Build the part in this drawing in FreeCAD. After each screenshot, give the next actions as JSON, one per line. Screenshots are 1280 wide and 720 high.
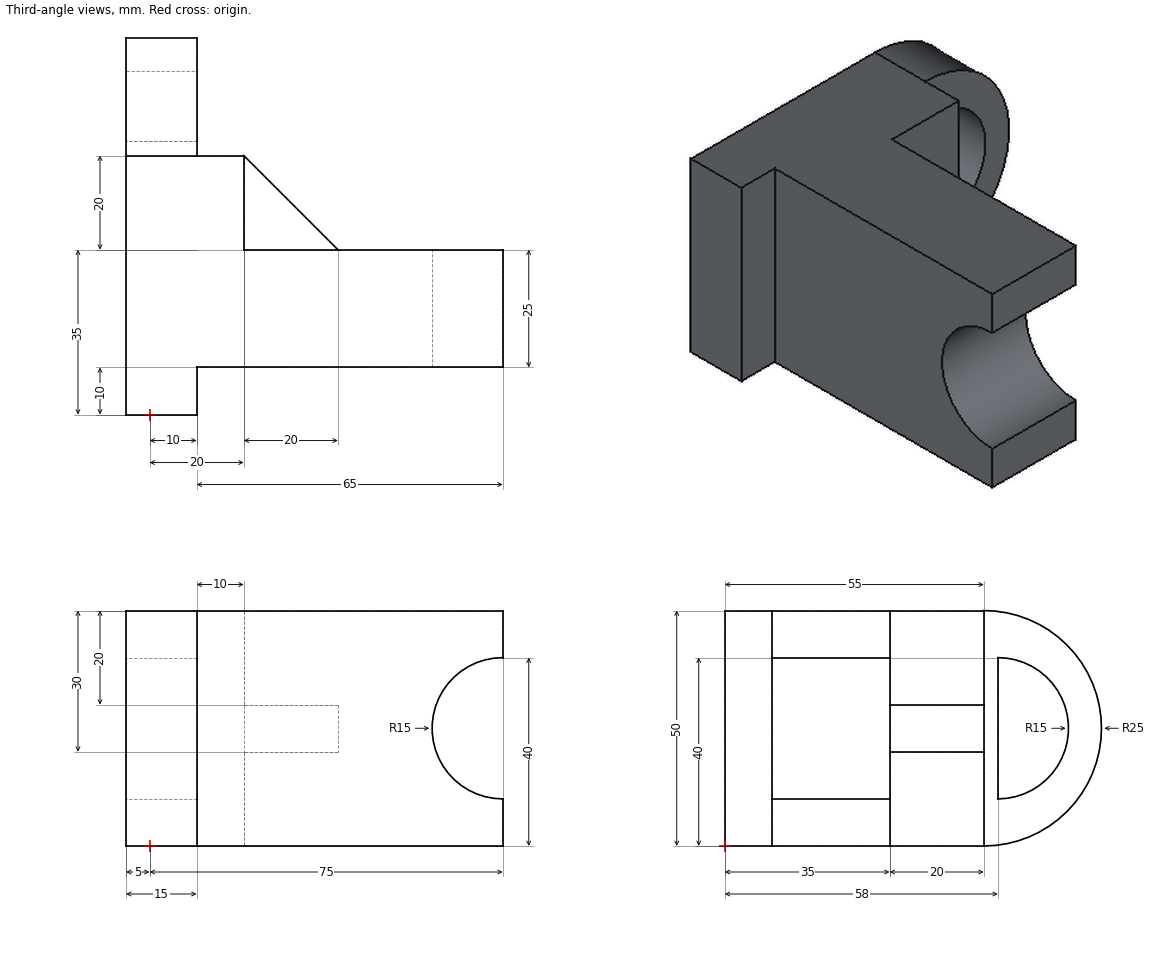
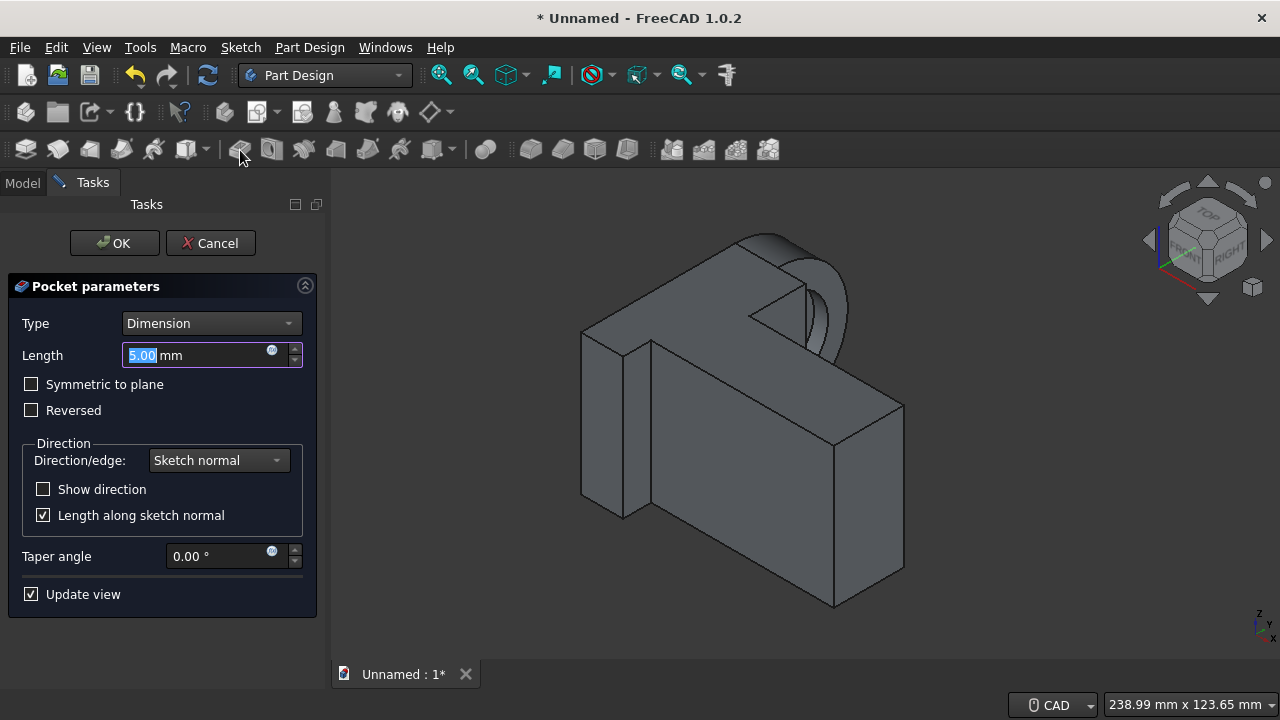
{"action": "type", "text": "15"}
{"action": "key", "text": "Tab"}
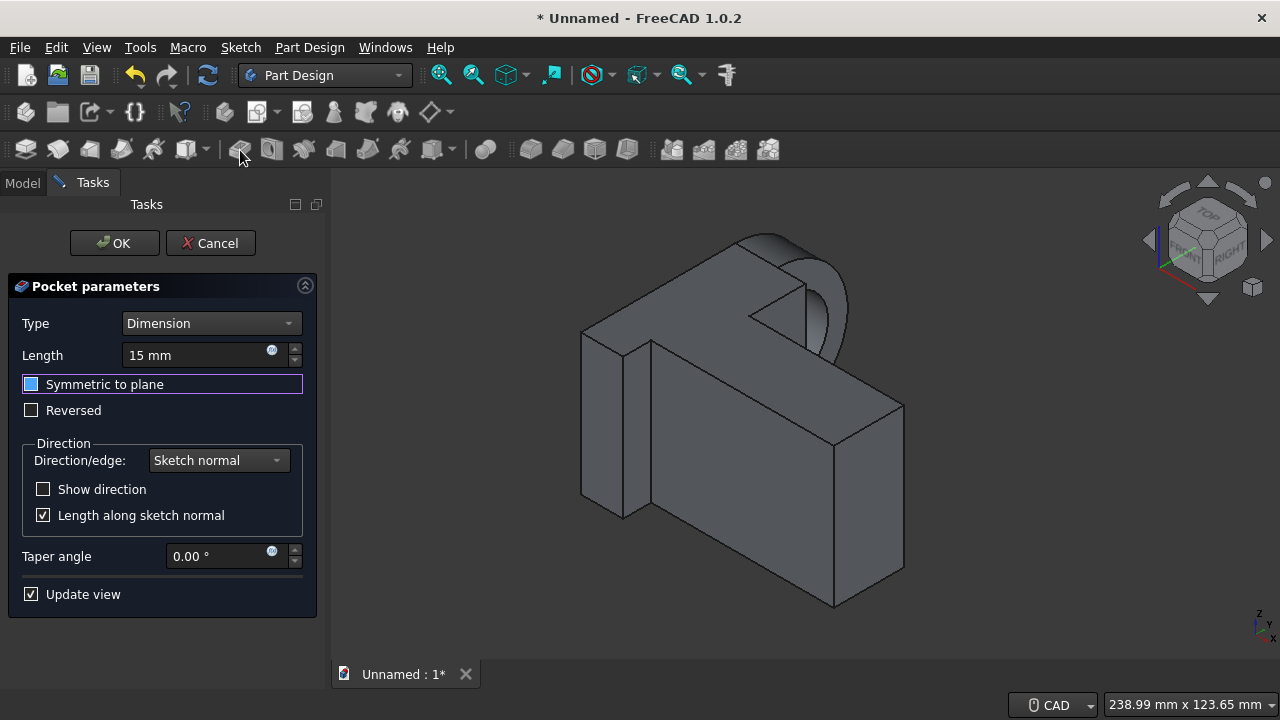
{"action": "left_click", "coordinate": [115, 243]}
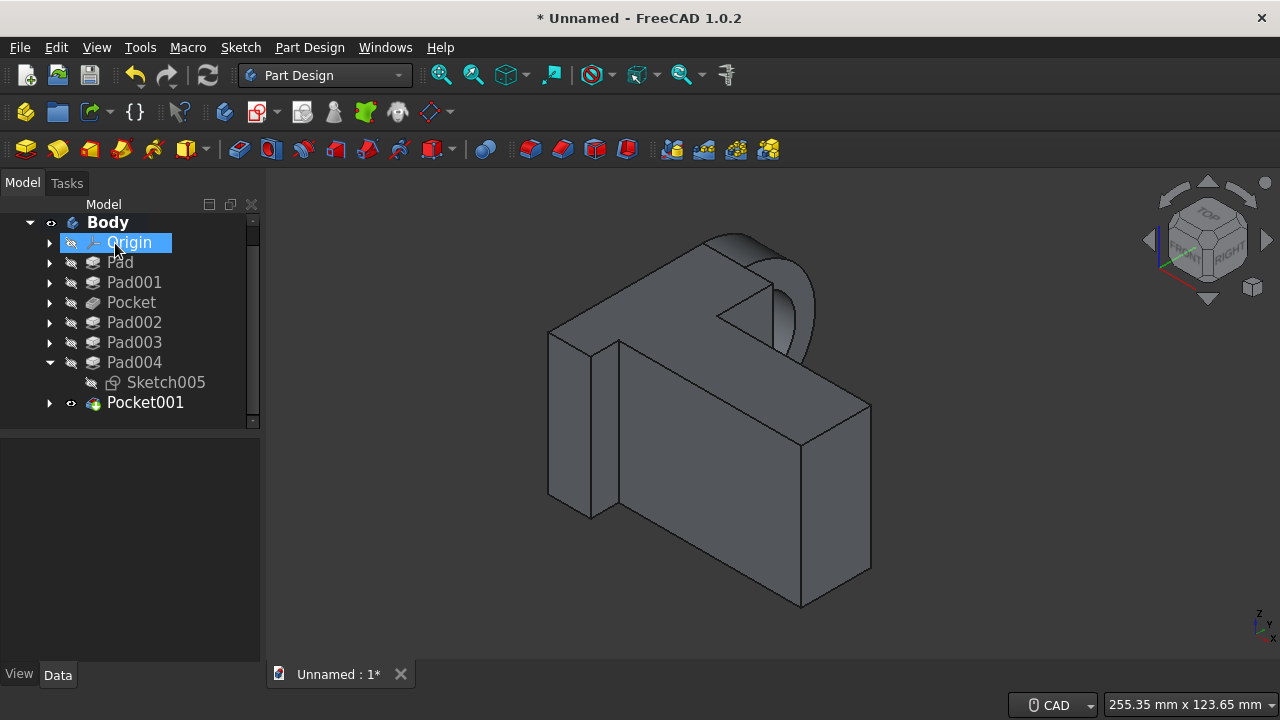
{"action": "key", "text": "4"}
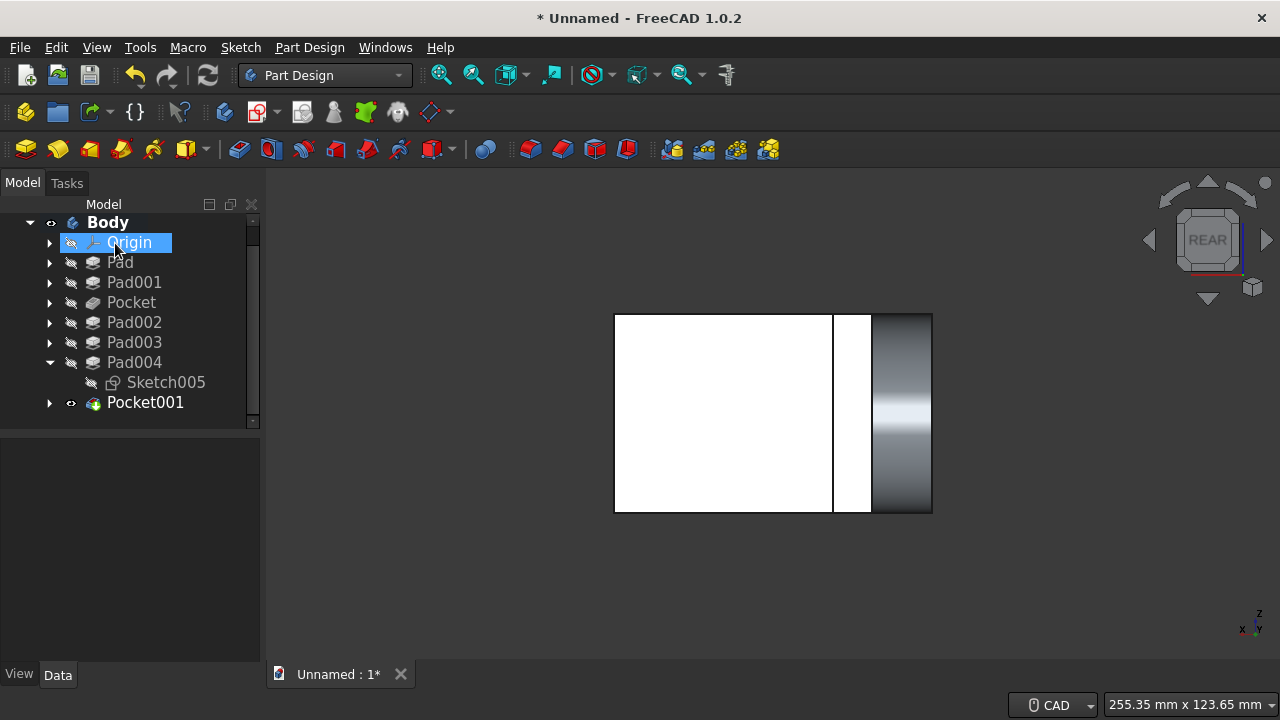
{"action": "left_click", "coordinate": [442, 76]}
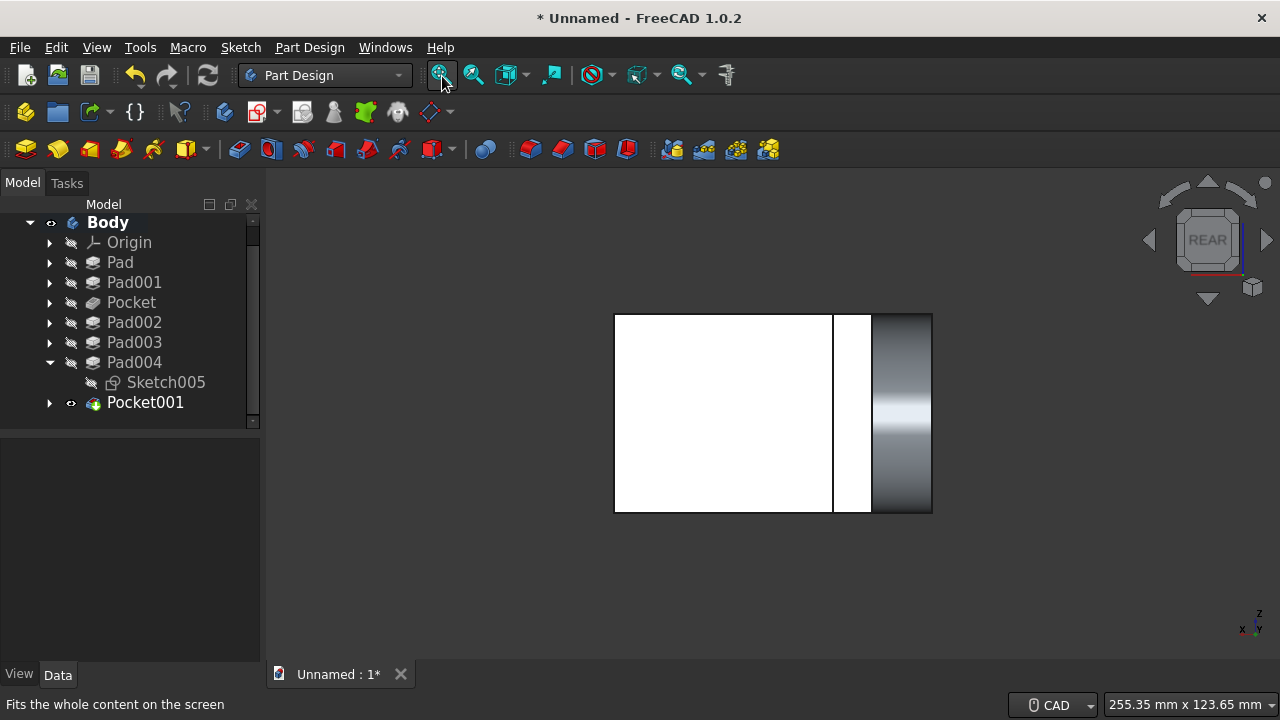
{"action": "left_click", "coordinate": [723, 413]}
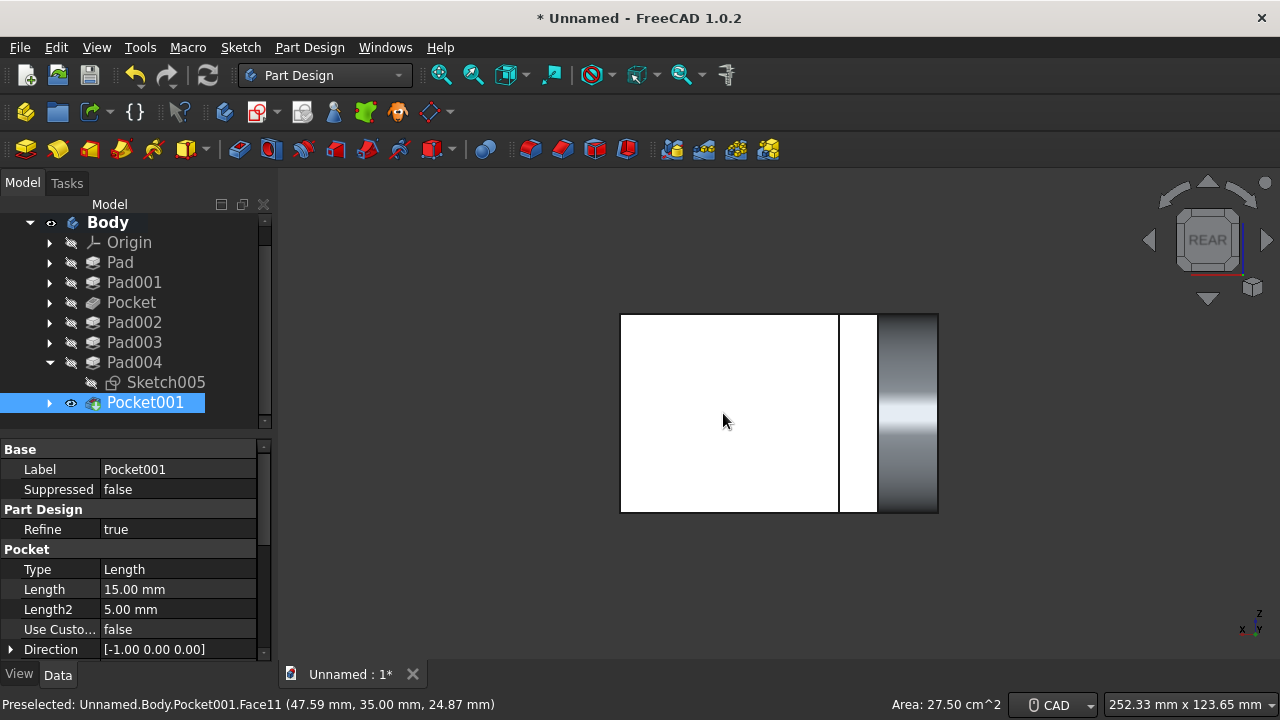
{"action": "left_click", "coordinate": [258, 112]}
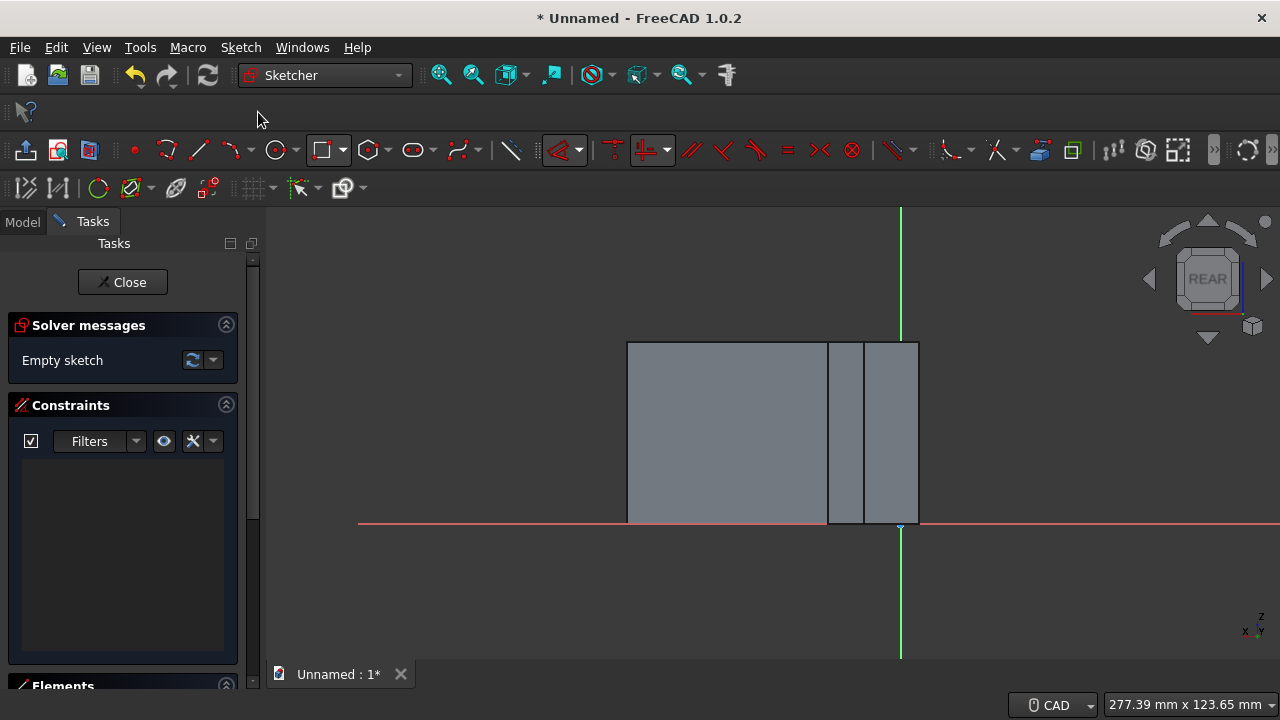
{"action": "scroll", "coordinate": [625, 433], "scroll_direction": "up", "scroll_amount": 5}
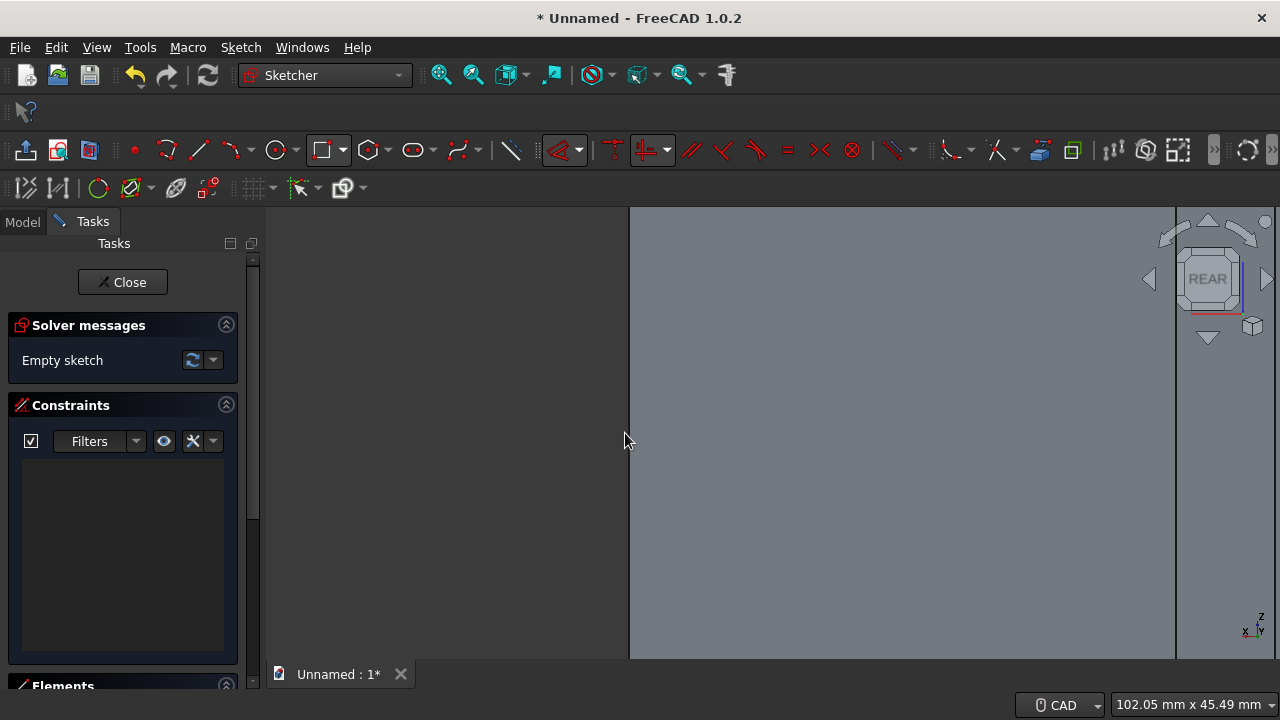
{"action": "left_click", "coordinate": [200, 150]}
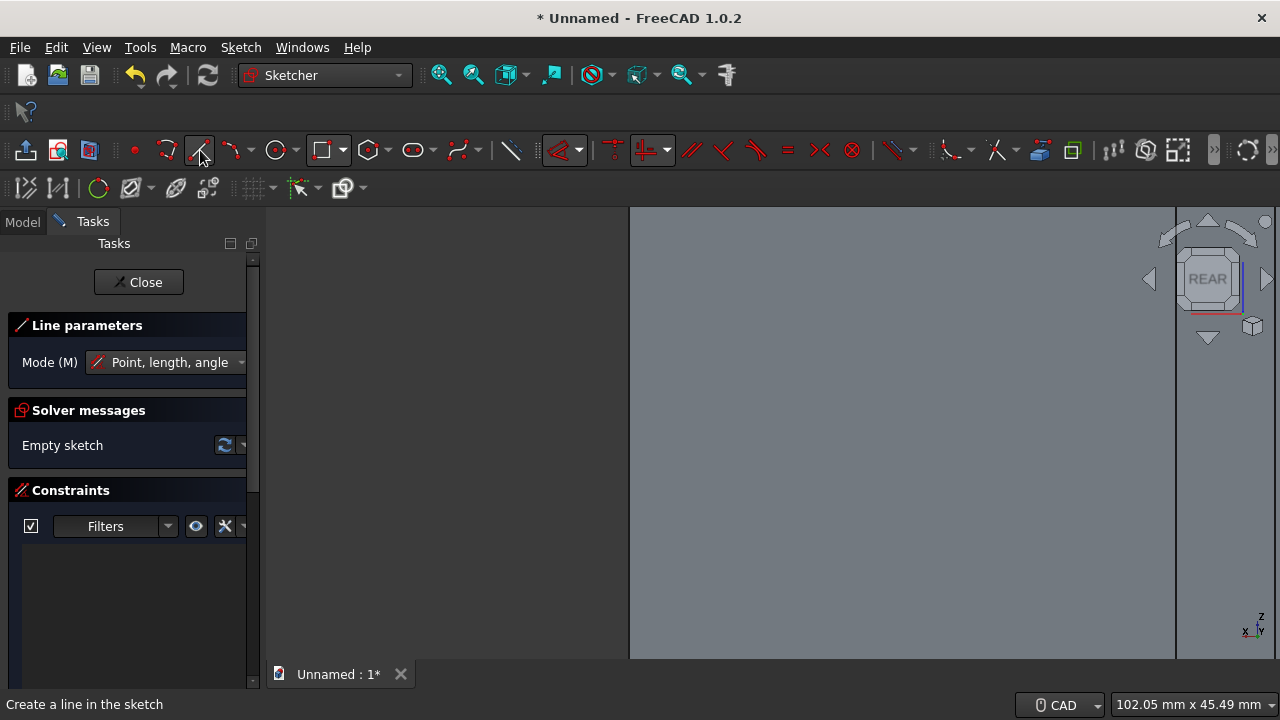
{"action": "left_click", "coordinate": [629, 283]}
{"action": "left_click", "coordinate": [629, 581]}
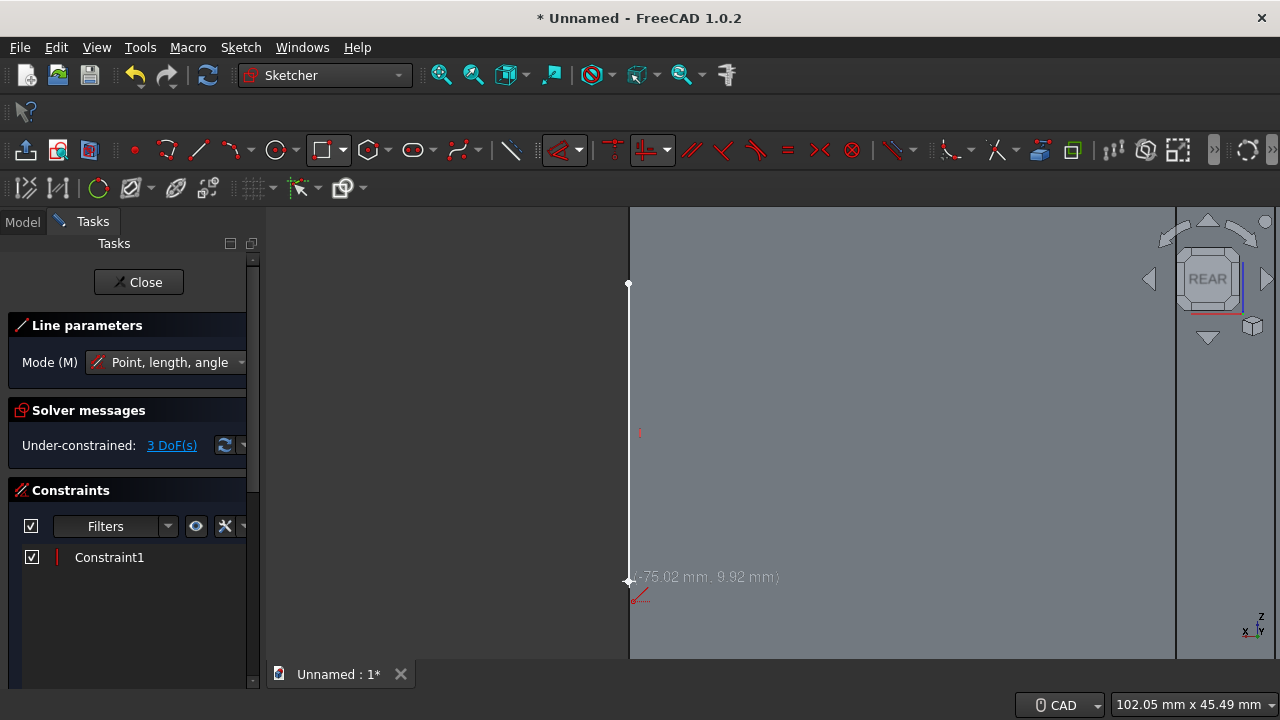
{"action": "left_click", "coordinate": [232, 150]}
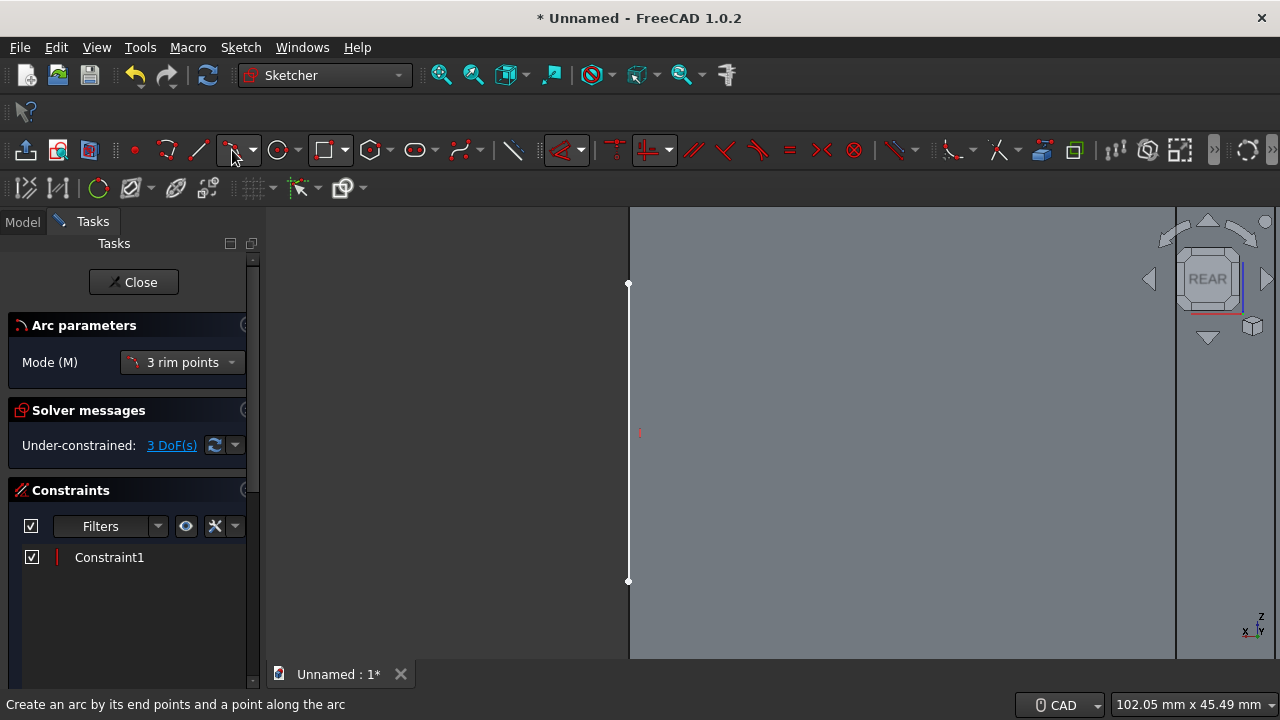
{"action": "left_click", "coordinate": [629, 582]}
{"action": "left_click", "coordinate": [629, 284]}
{"action": "left_click", "coordinate": [778, 432]}
{"action": "key", "text": "Escape"}